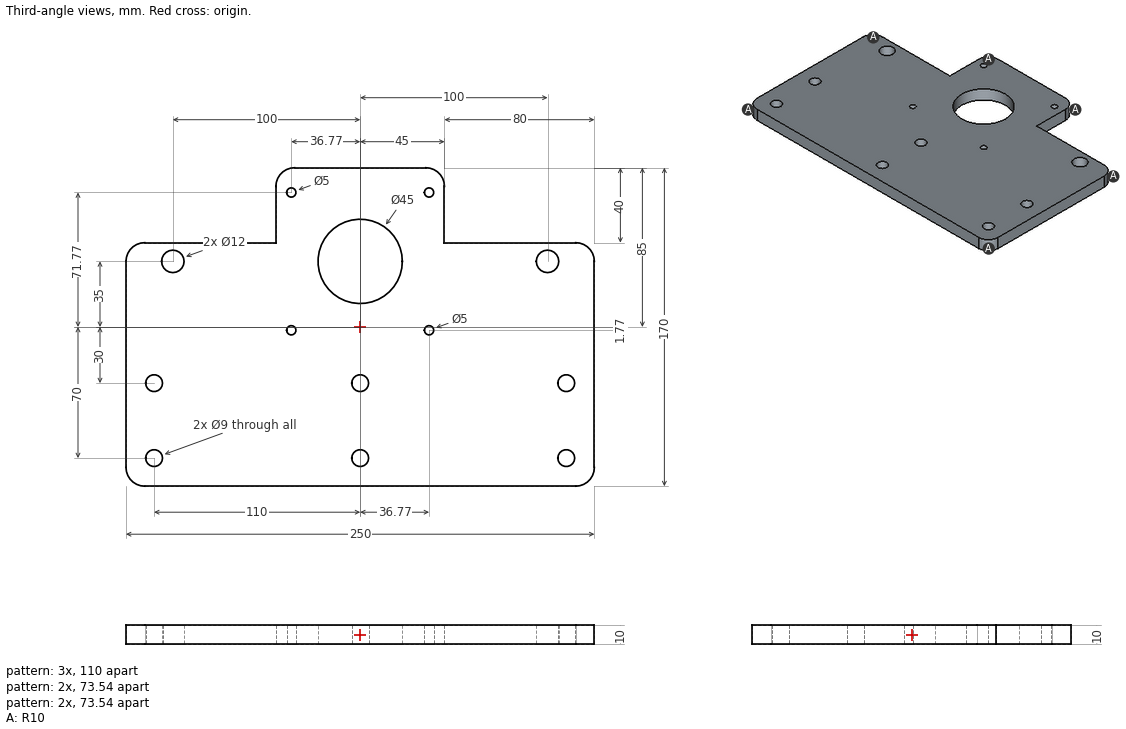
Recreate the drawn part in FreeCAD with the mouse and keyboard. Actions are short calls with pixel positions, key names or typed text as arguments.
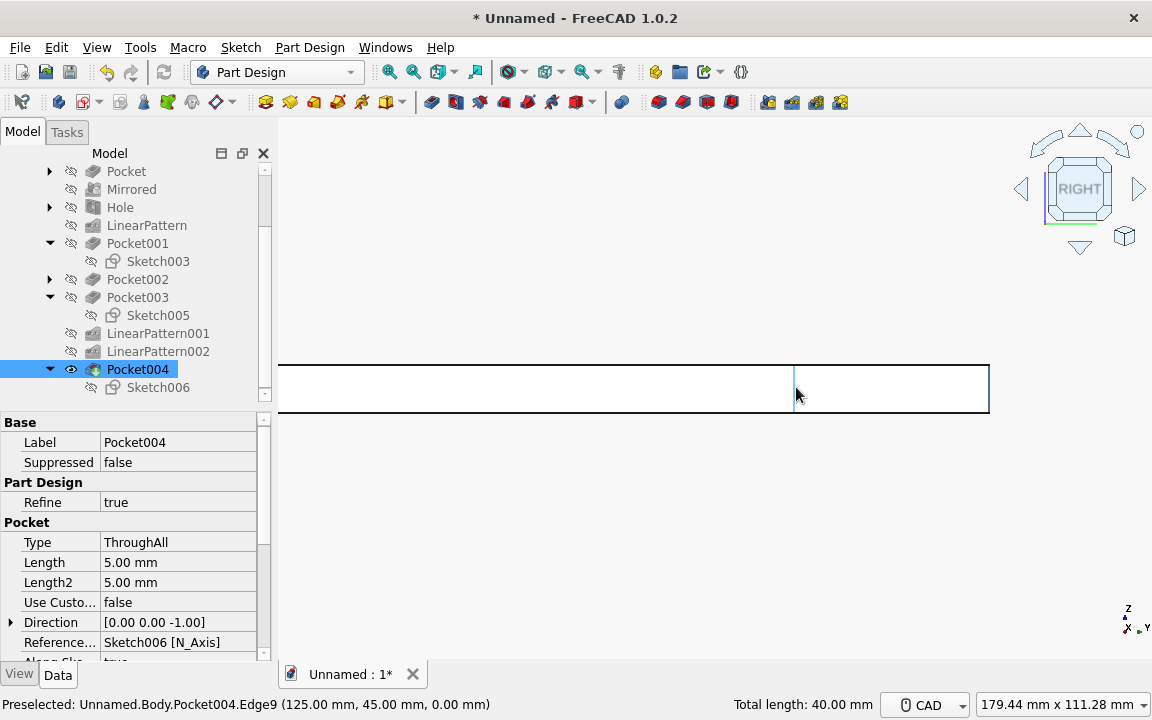
key(v)
key(f)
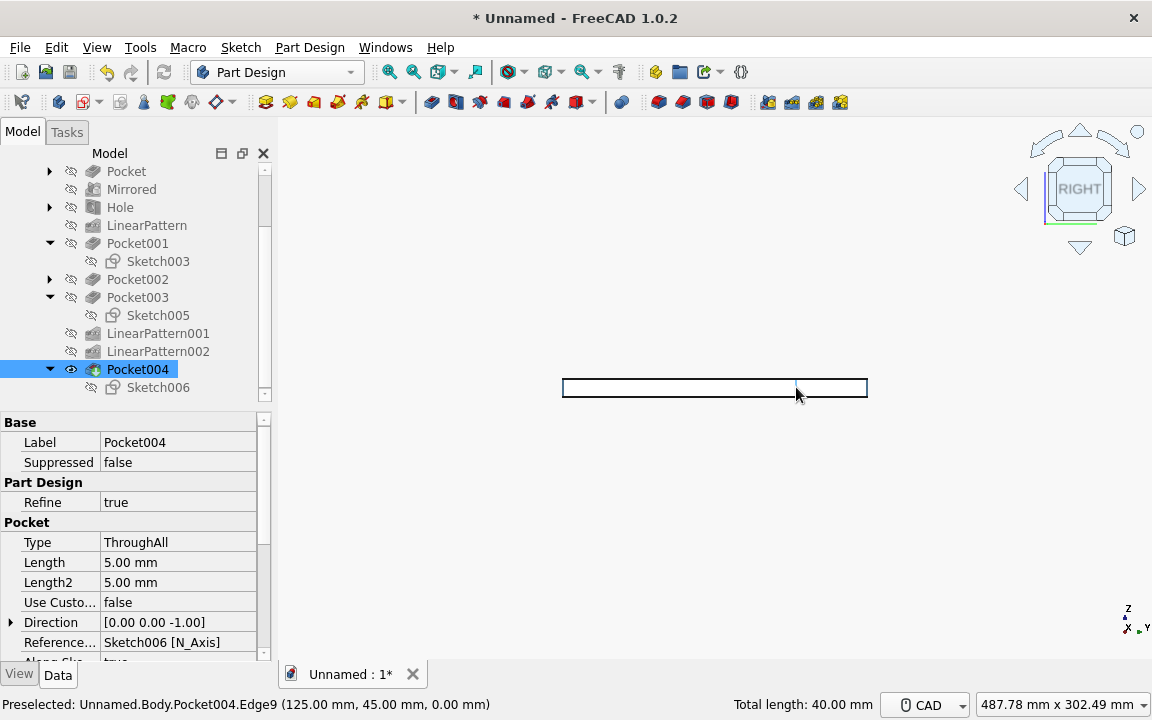
key(5)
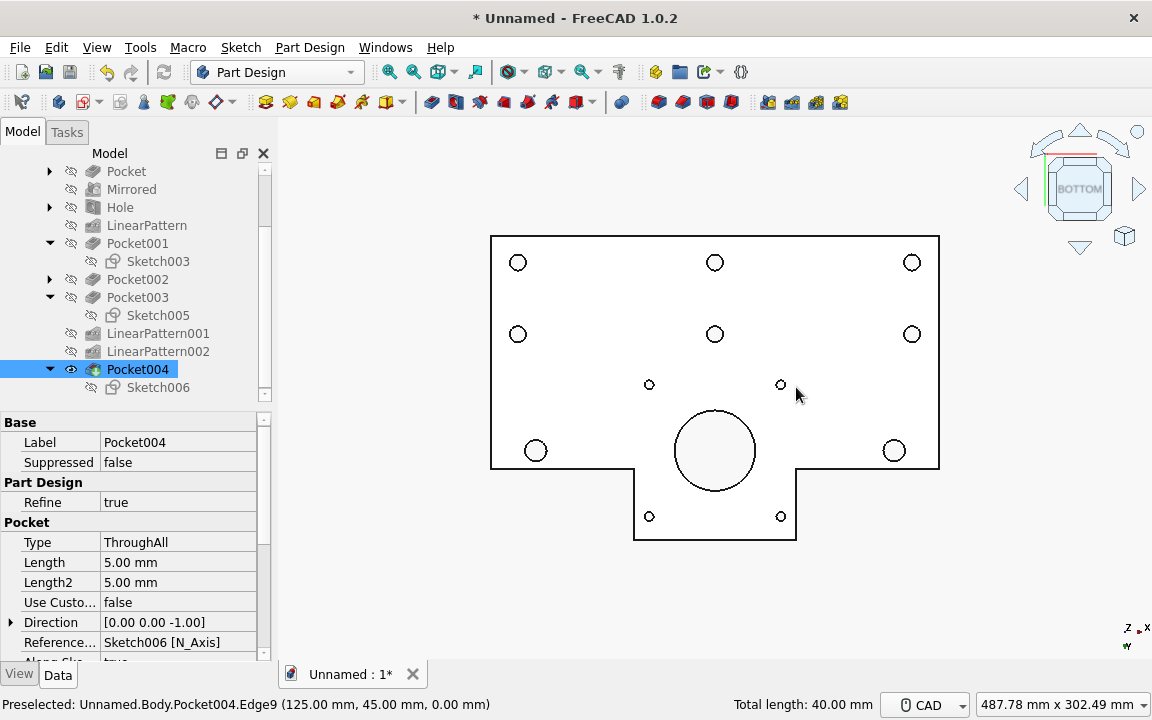
scroll(491, 468, up, 5)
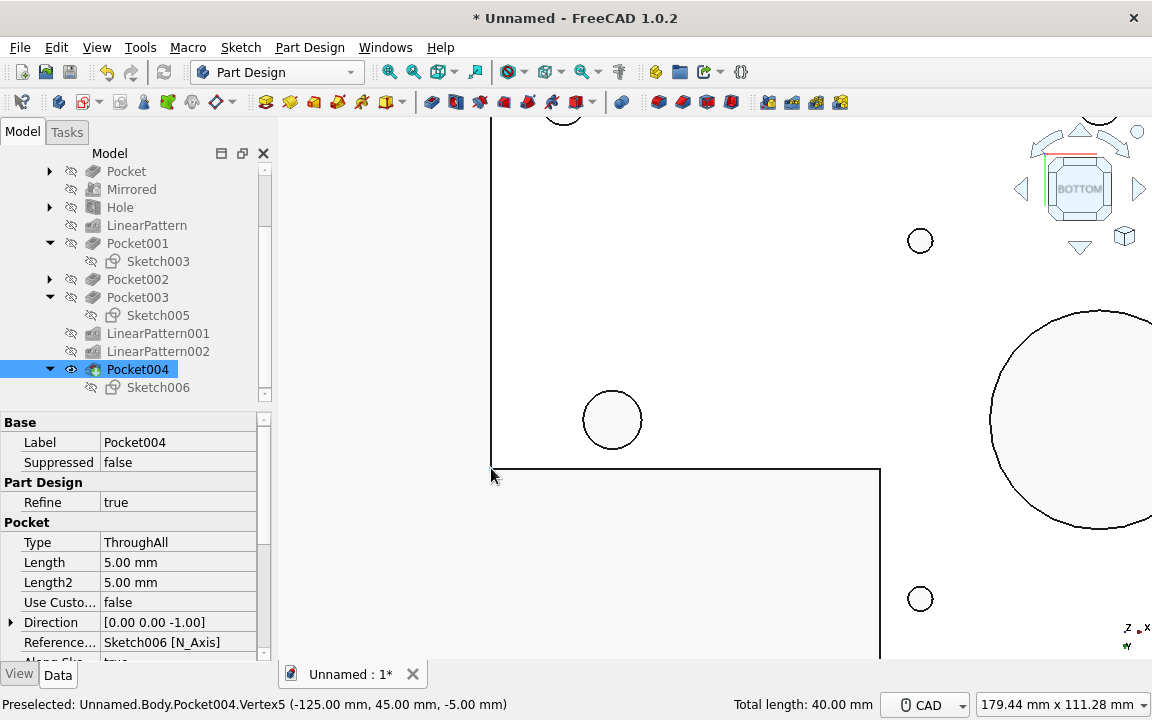
key(v)
key(f)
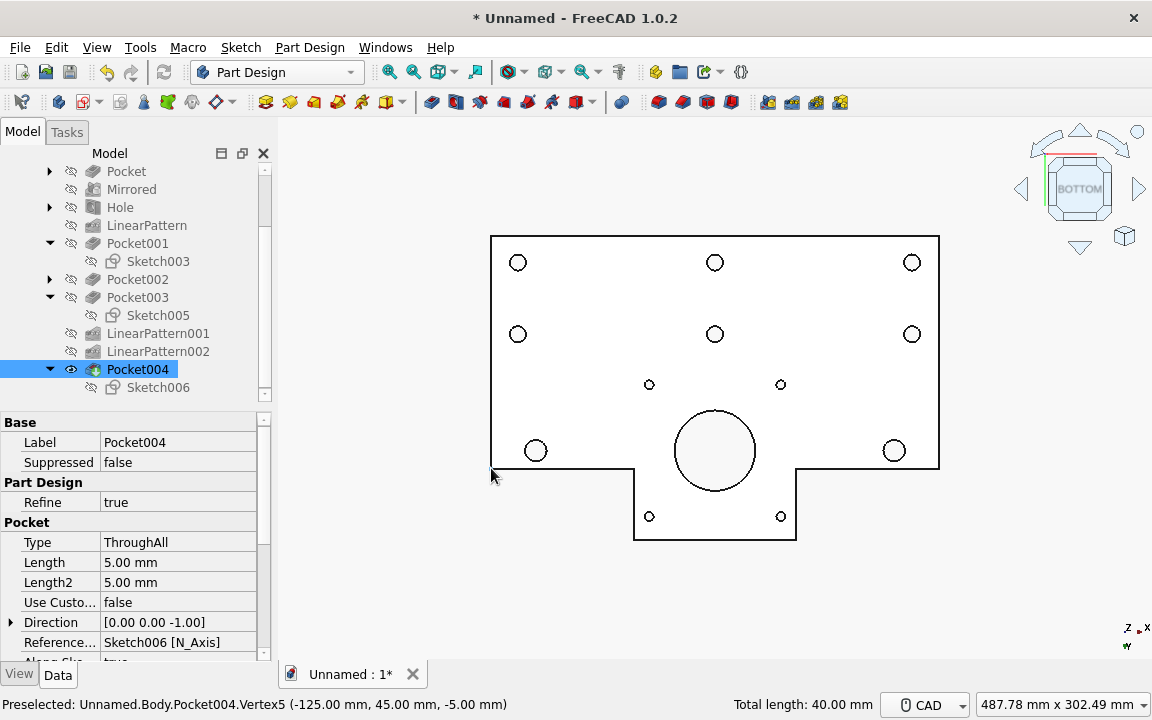
key(4)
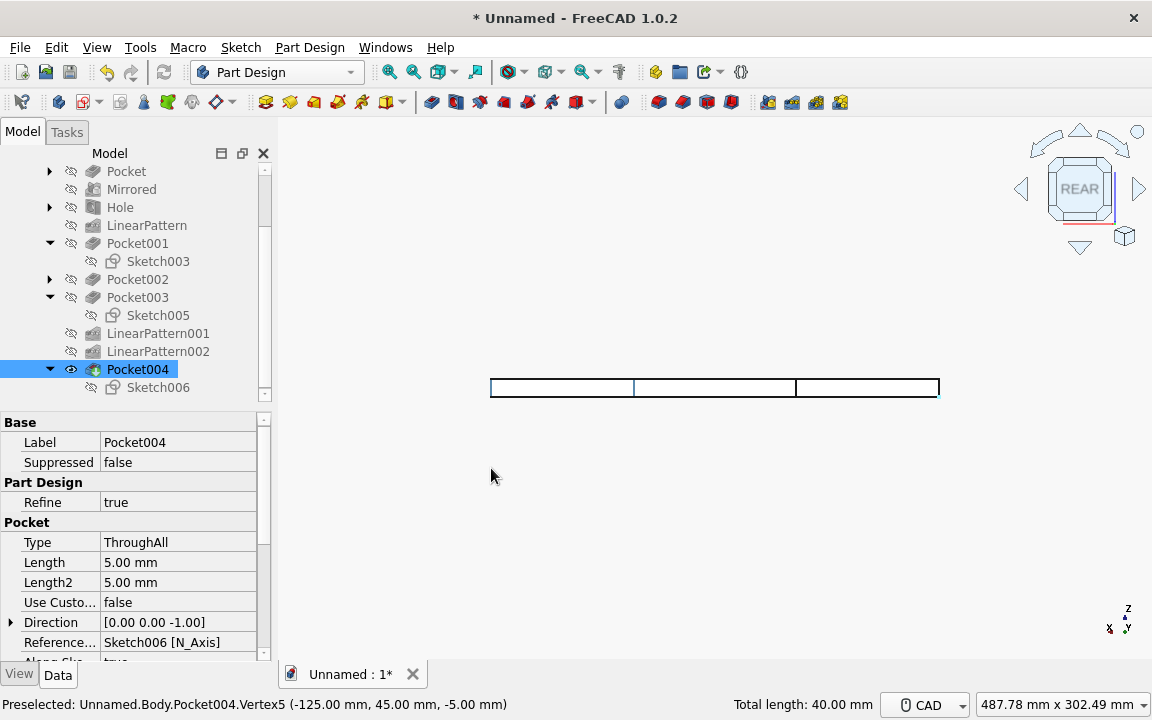
click(939, 387, ctrl)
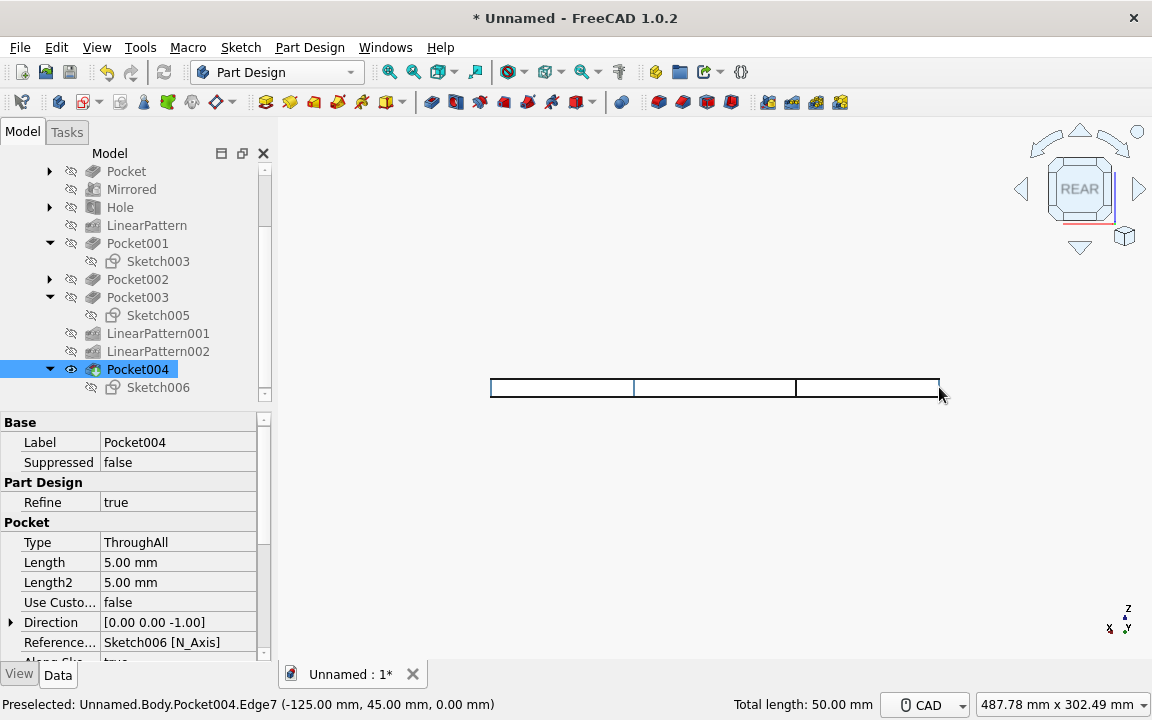
click(796, 387, ctrl)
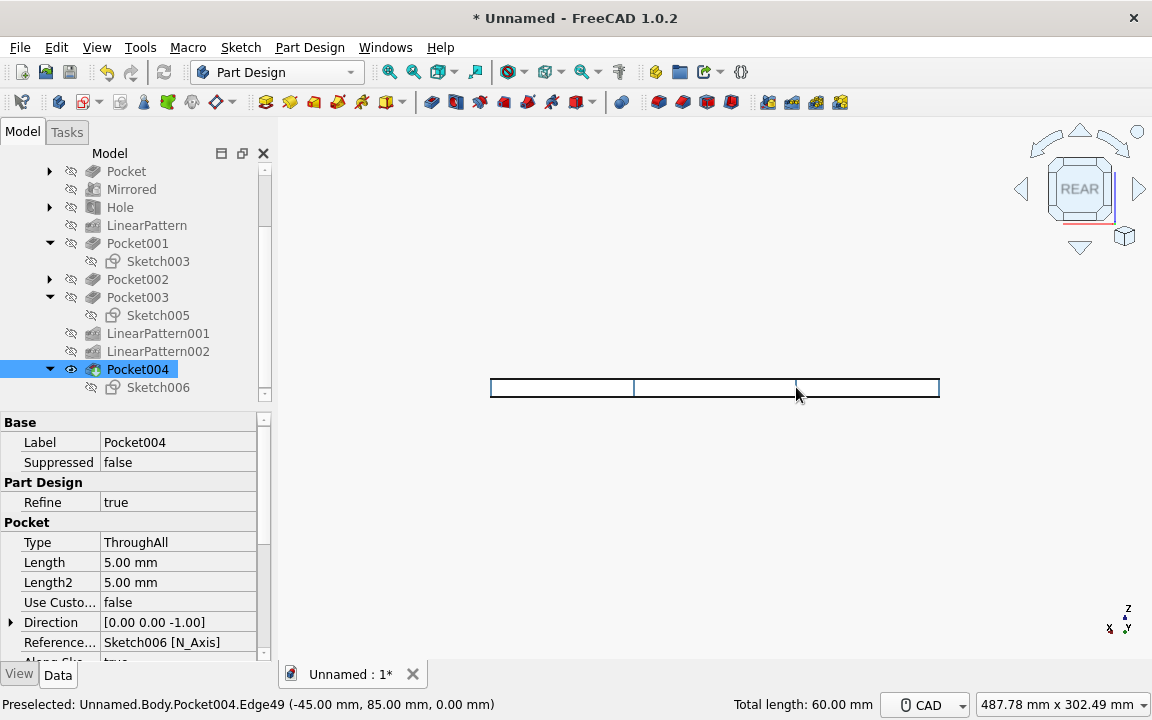
click(660, 102)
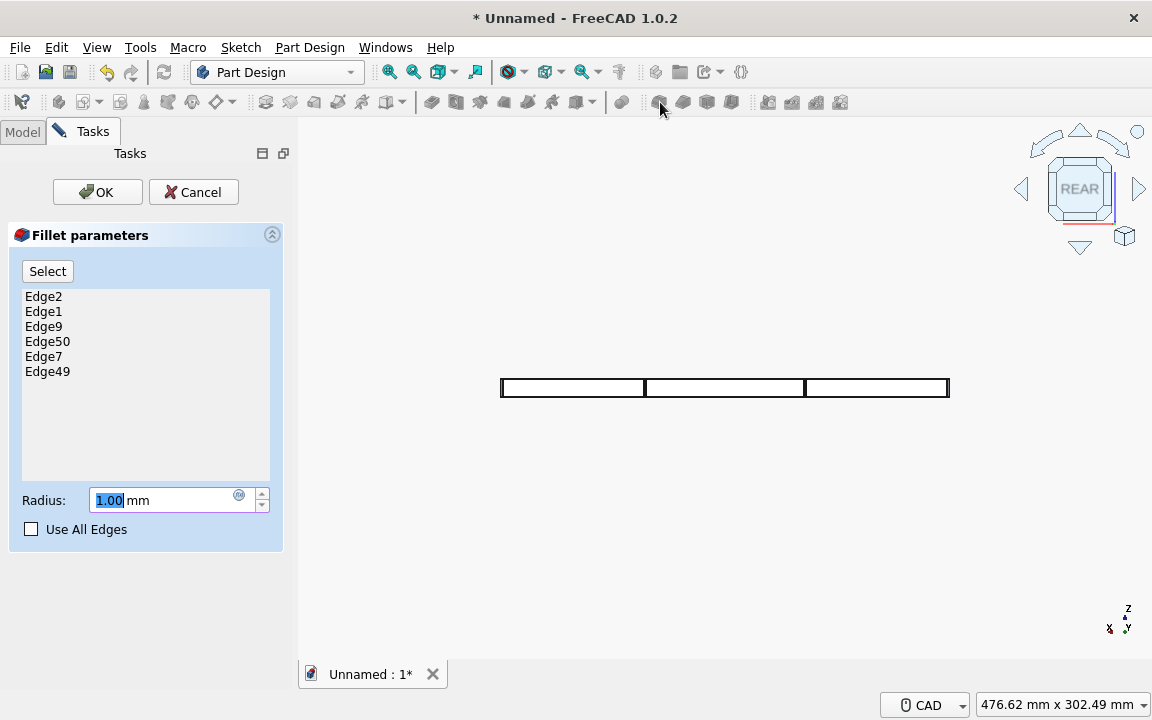
text(10)
key(Tab)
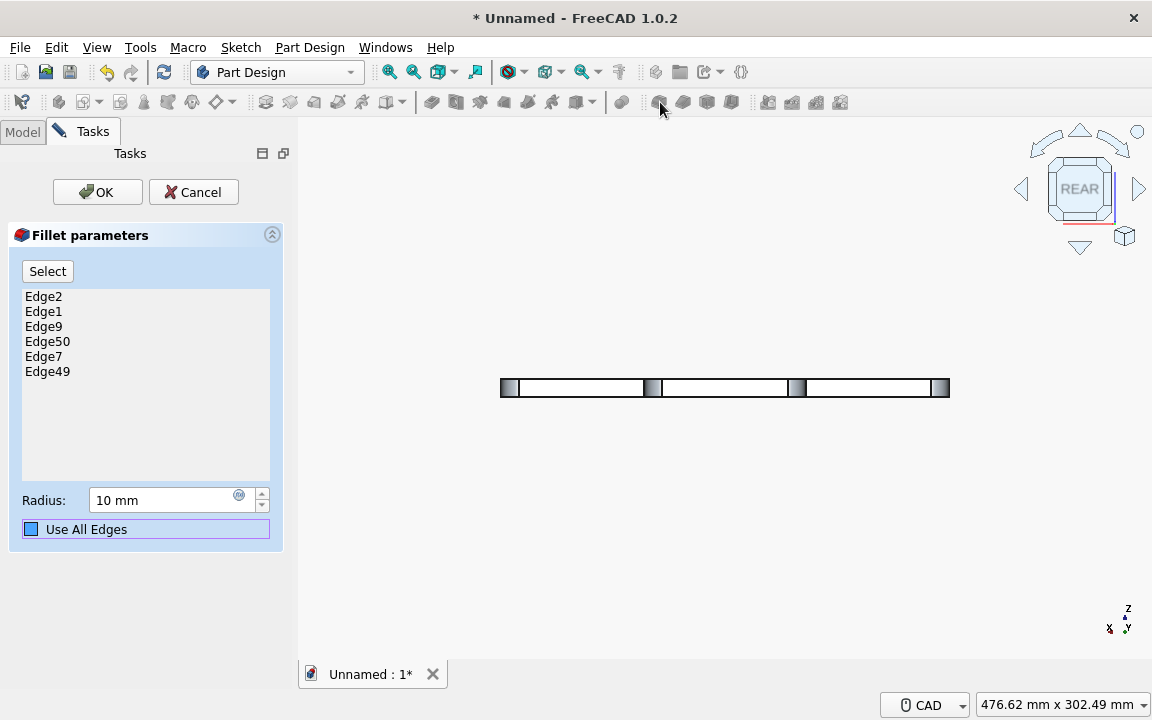
click(98, 192)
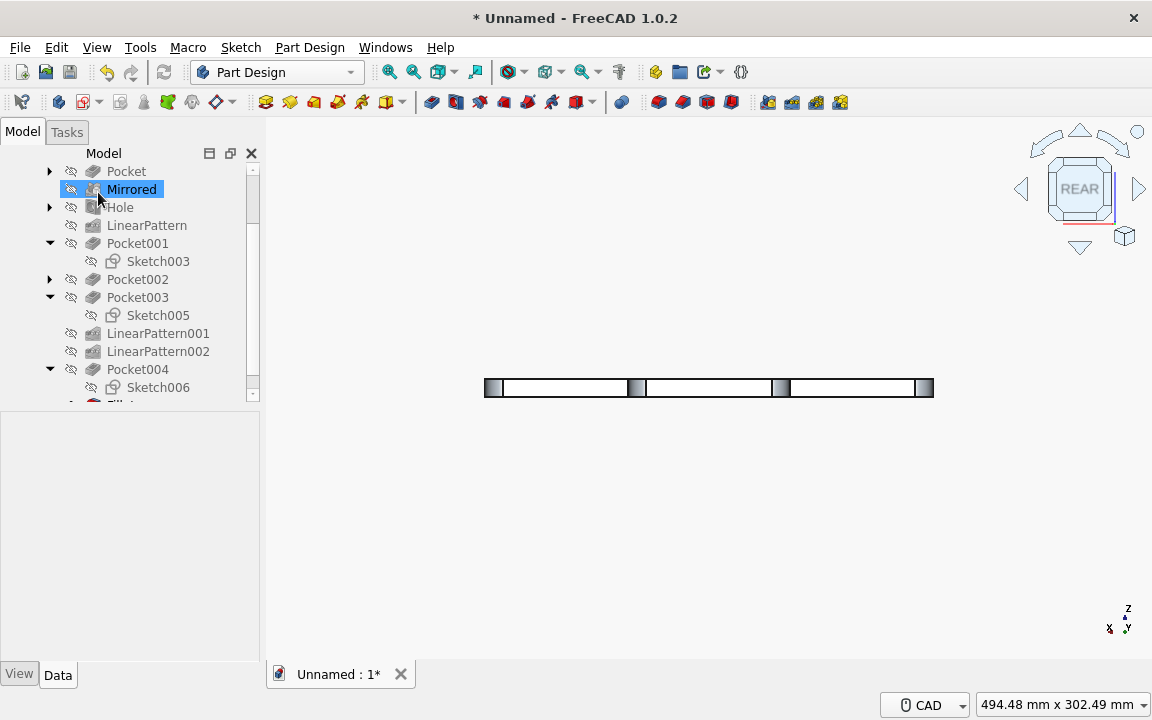
key(0)